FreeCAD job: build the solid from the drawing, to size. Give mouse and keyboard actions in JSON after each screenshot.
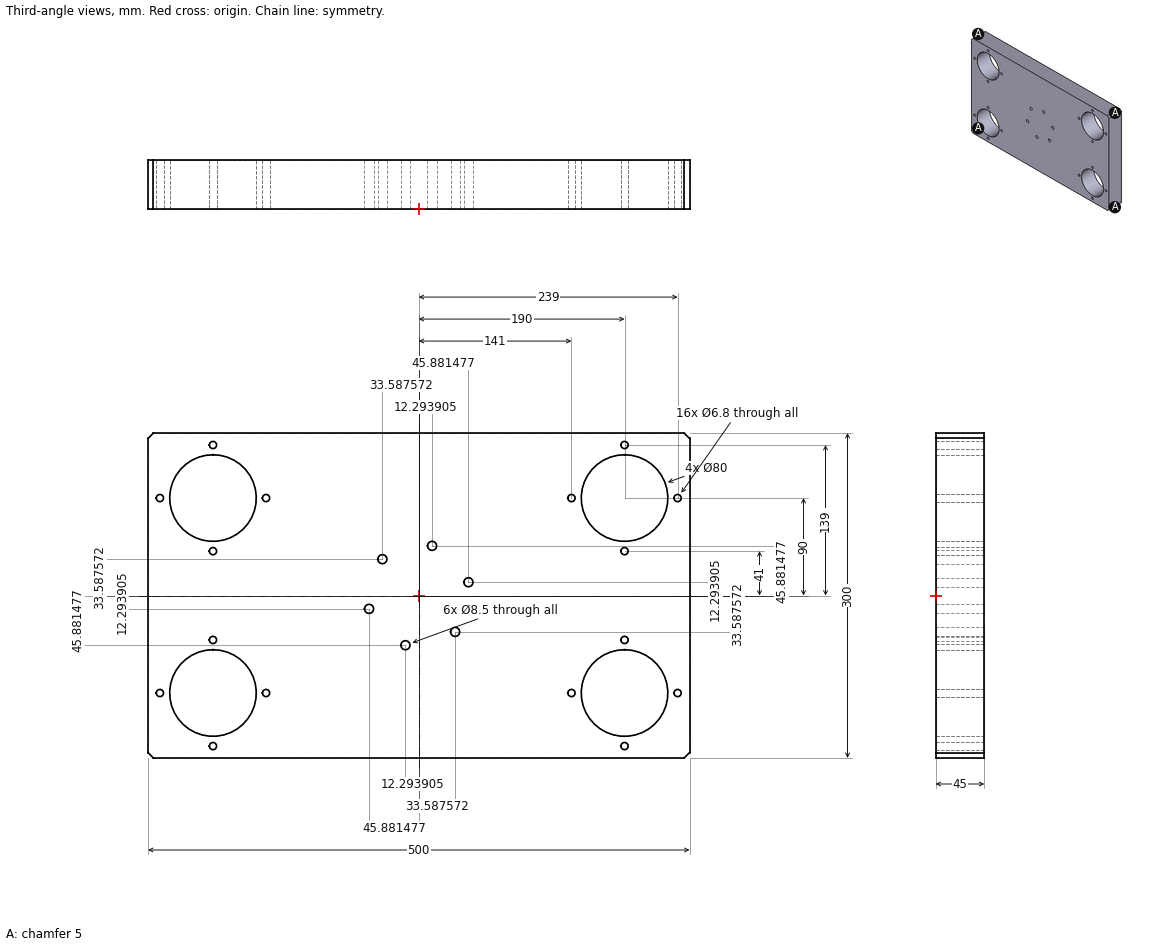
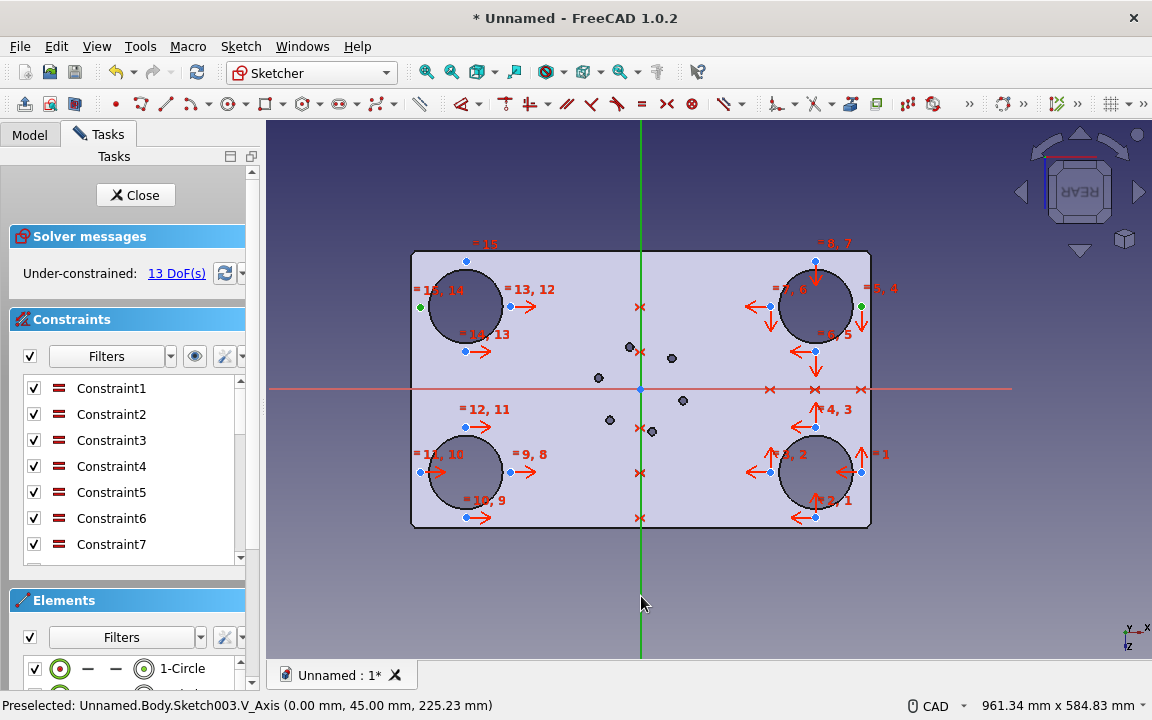
{"action": "left_click", "coordinate": [667, 104]}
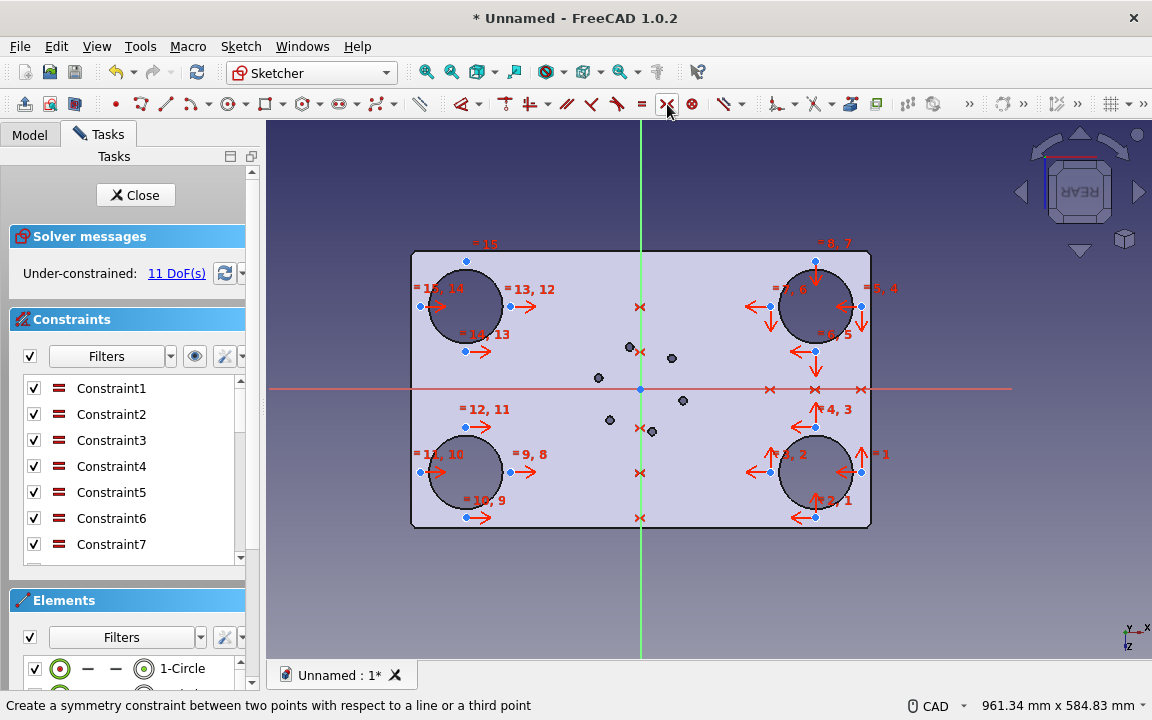
{"action": "left_click", "coordinate": [816, 261]}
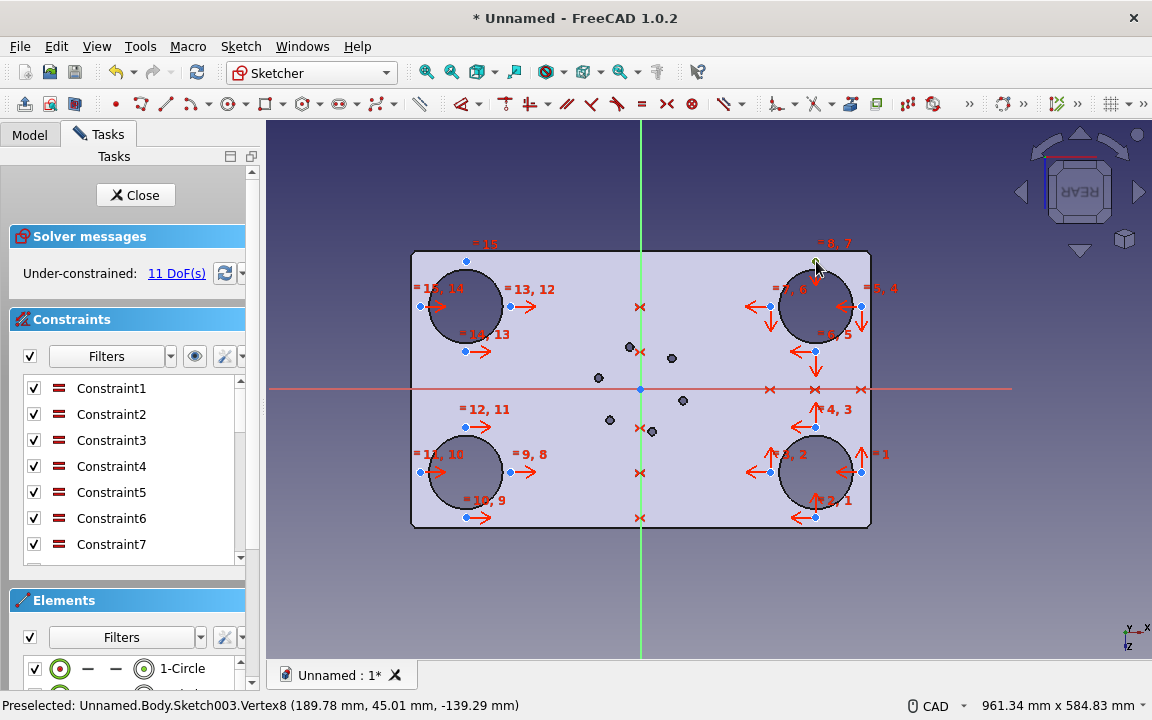
{"action": "left_click", "coordinate": [466, 262]}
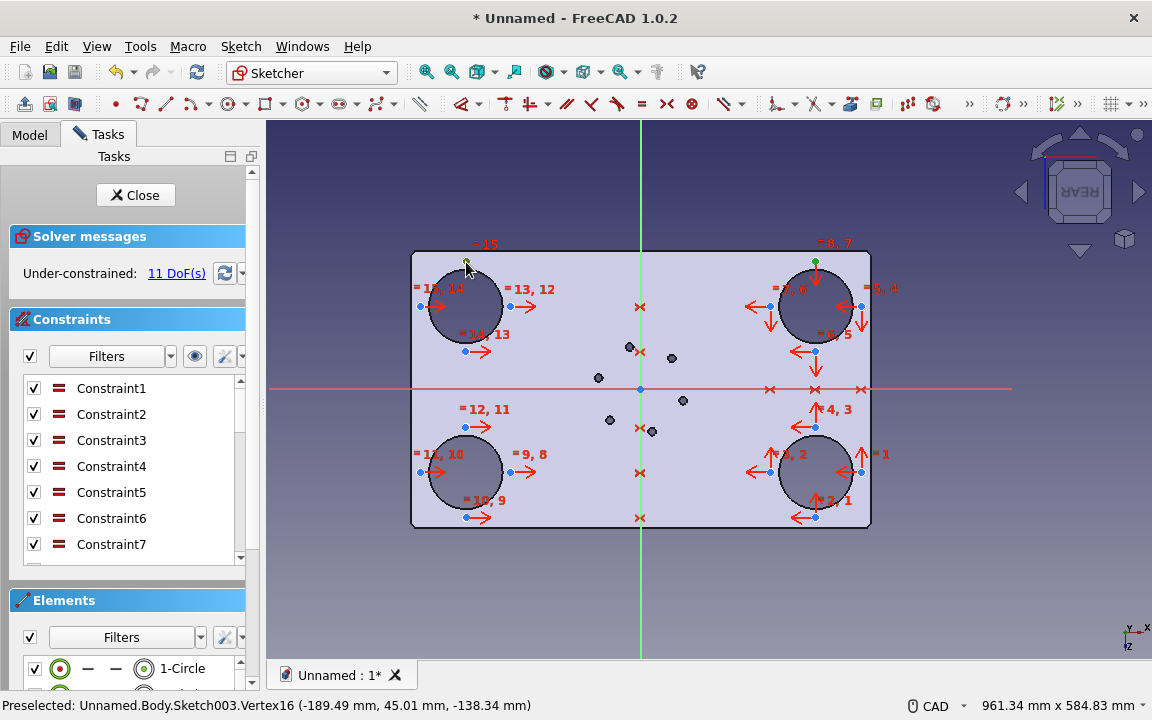
{"action": "left_click", "coordinate": [641, 596]}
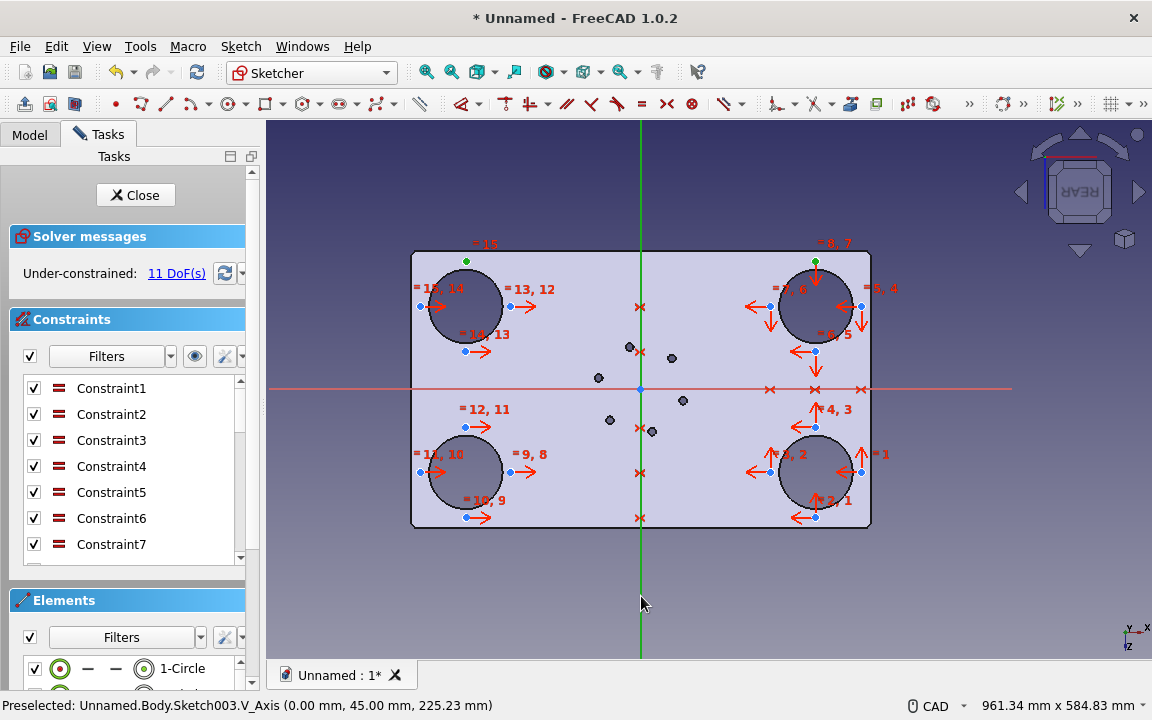
{"action": "left_click", "coordinate": [667, 104]}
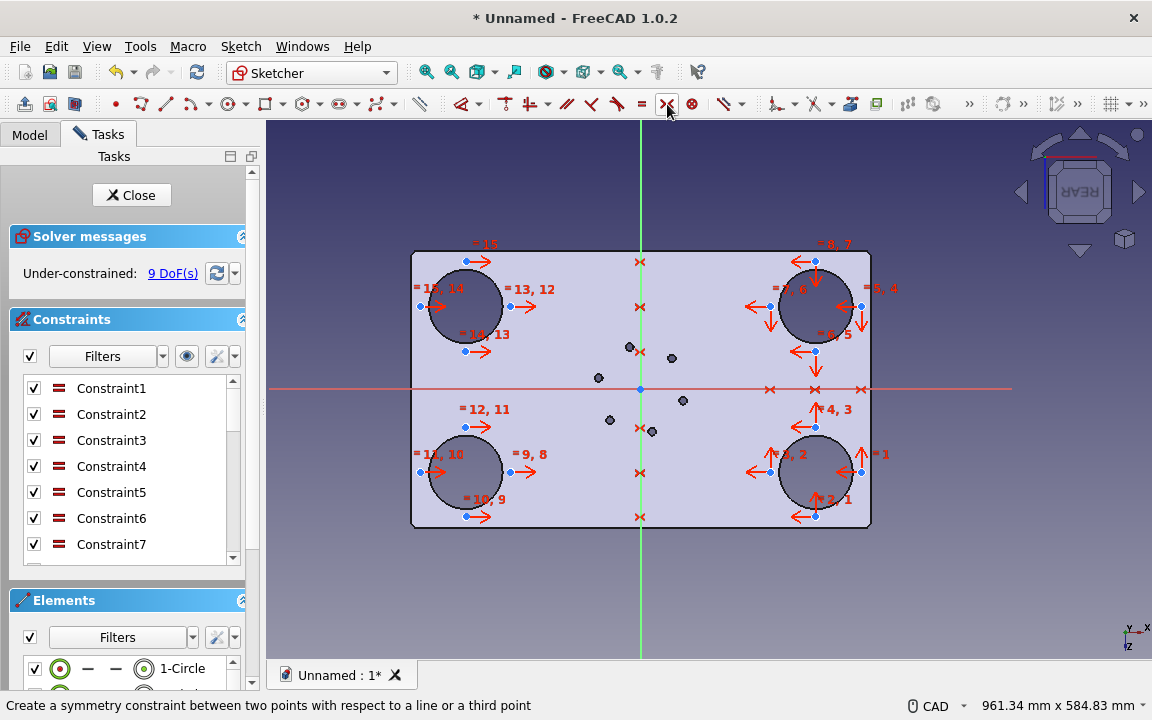
{"action": "left_click", "coordinate": [460, 104]}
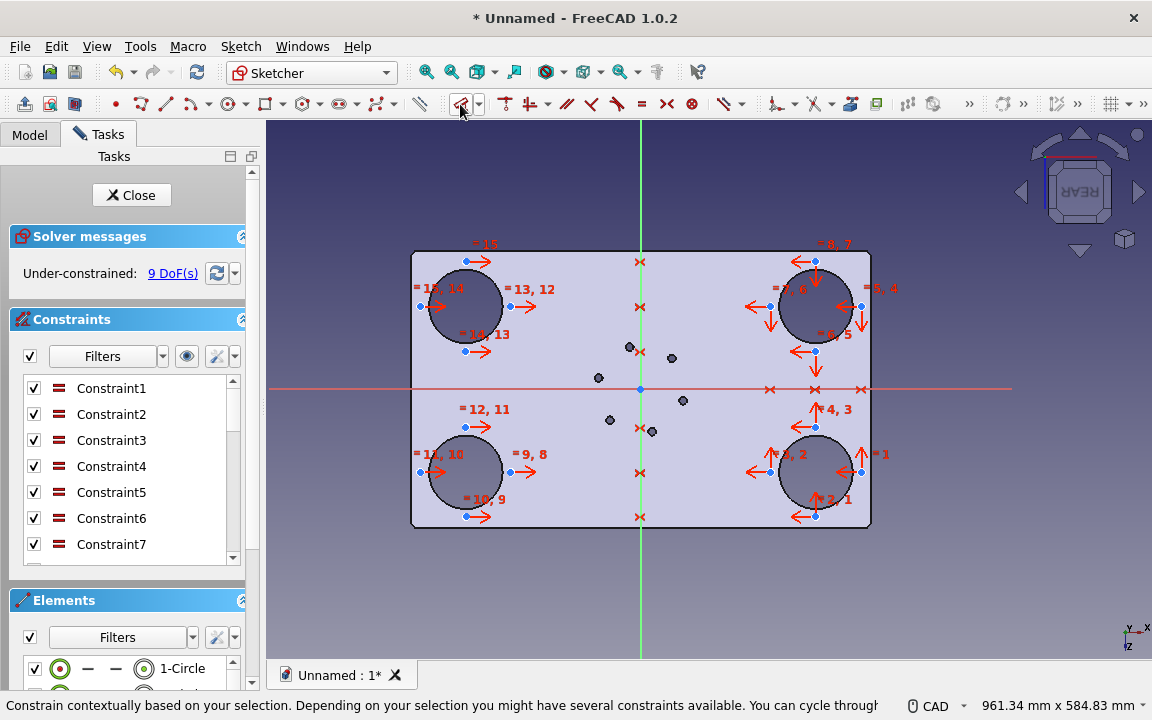
{"action": "scroll", "coordinate": [864, 470], "scroll_direction": "up", "scroll_amount": 10}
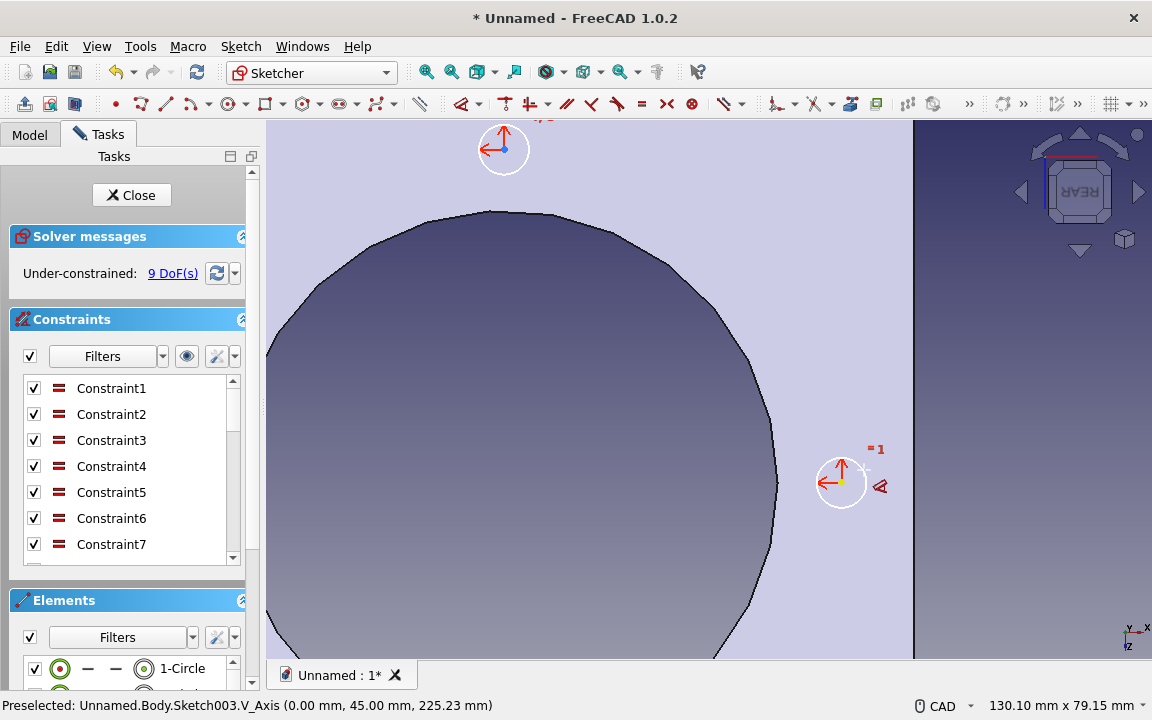
{"action": "left_click", "coordinate": [859, 465]}
{"action": "left_click", "coordinate": [881, 442]}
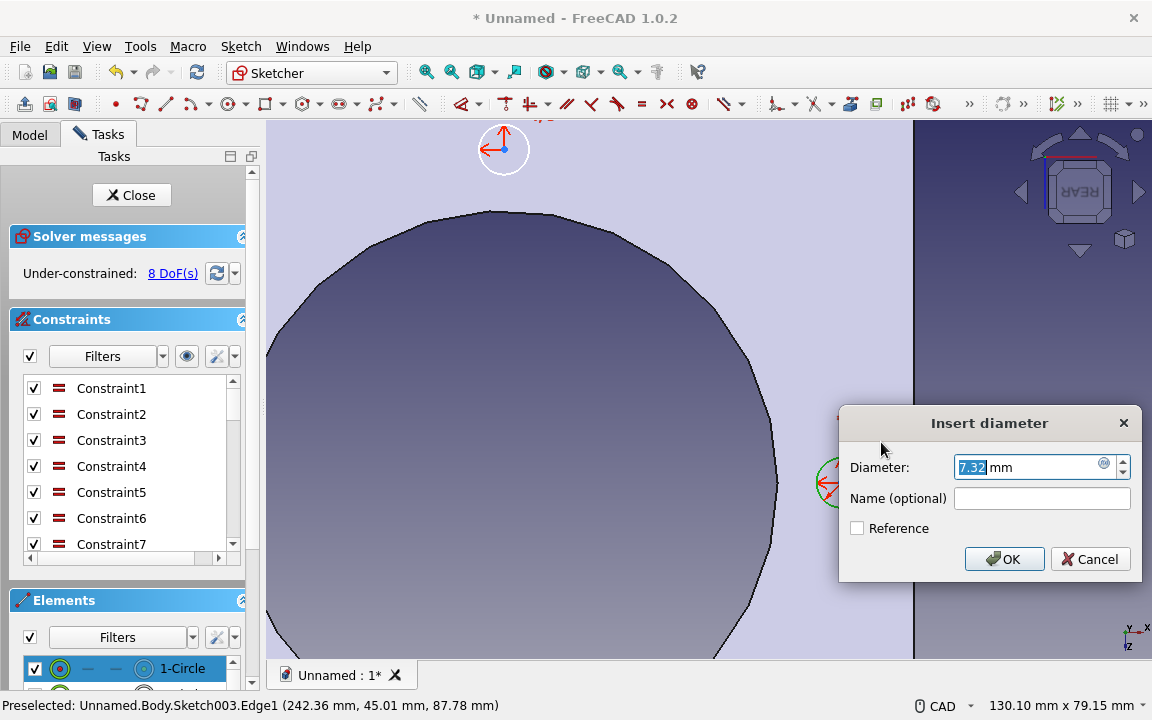
{"action": "type", "text": "6.8"}
{"action": "key", "text": "Return"}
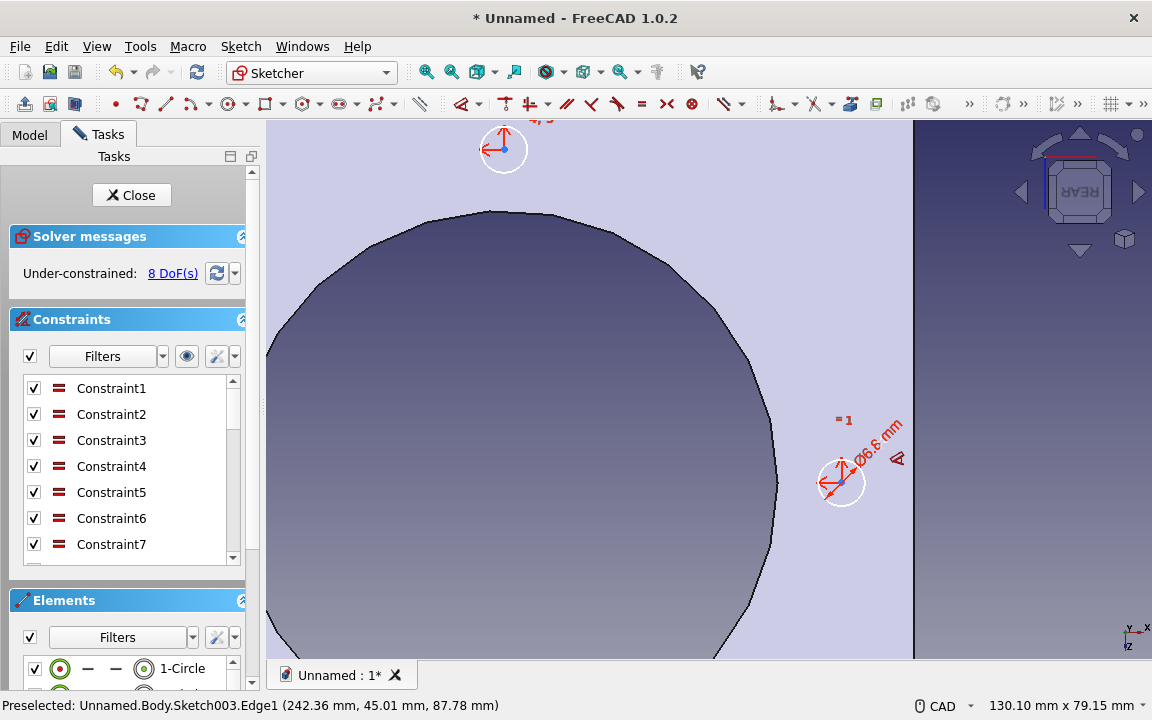
{"action": "scroll", "coordinate": [864, 471], "scroll_direction": "down", "scroll_amount": 10}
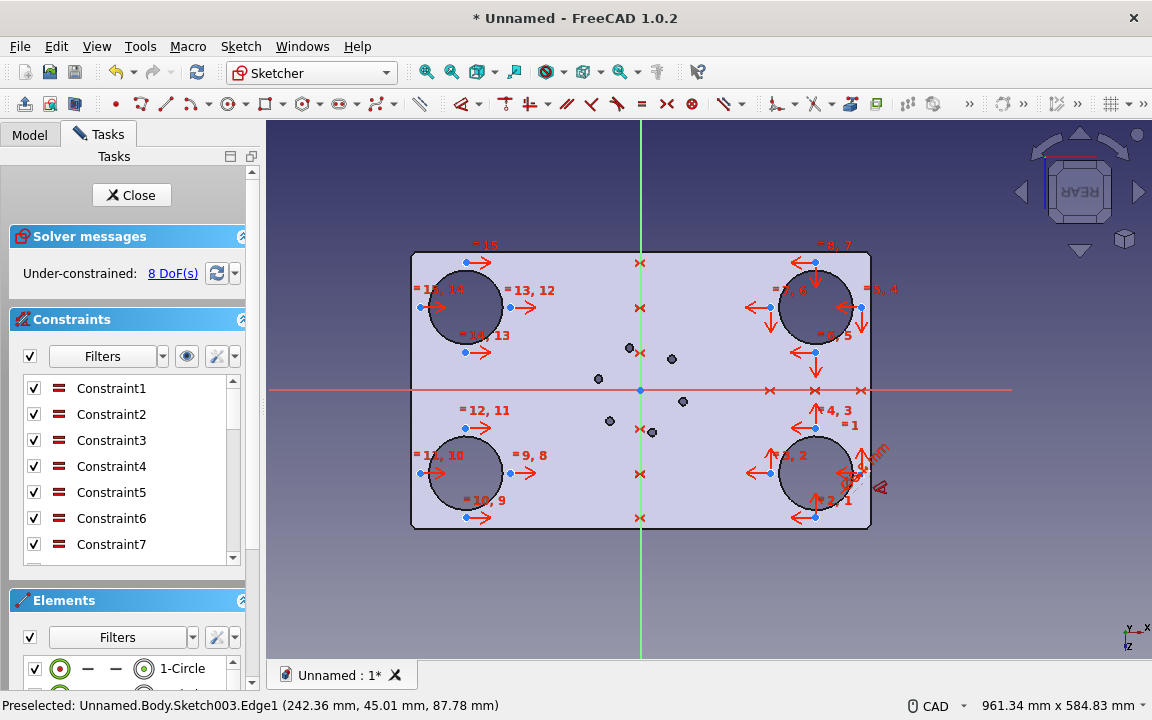
{"action": "left_click", "coordinate": [862, 473]}
{"action": "left_click", "coordinate": [896, 432]}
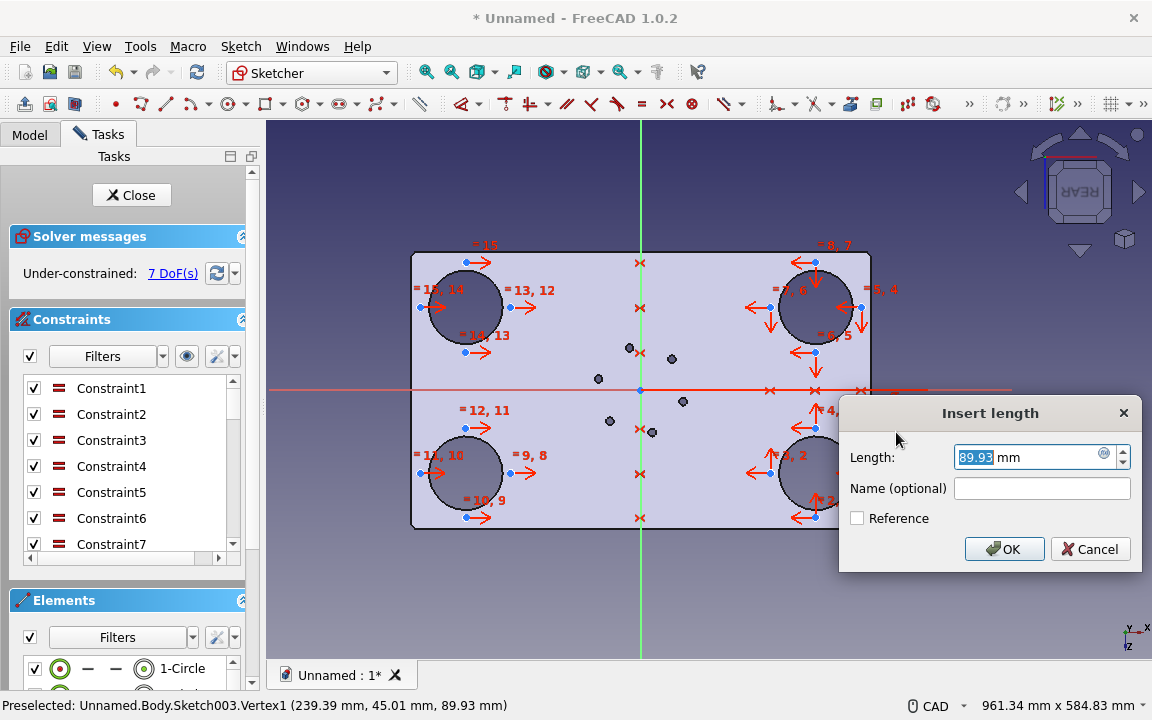
{"action": "type", "text": "90"}
{"action": "key", "text": "Return"}